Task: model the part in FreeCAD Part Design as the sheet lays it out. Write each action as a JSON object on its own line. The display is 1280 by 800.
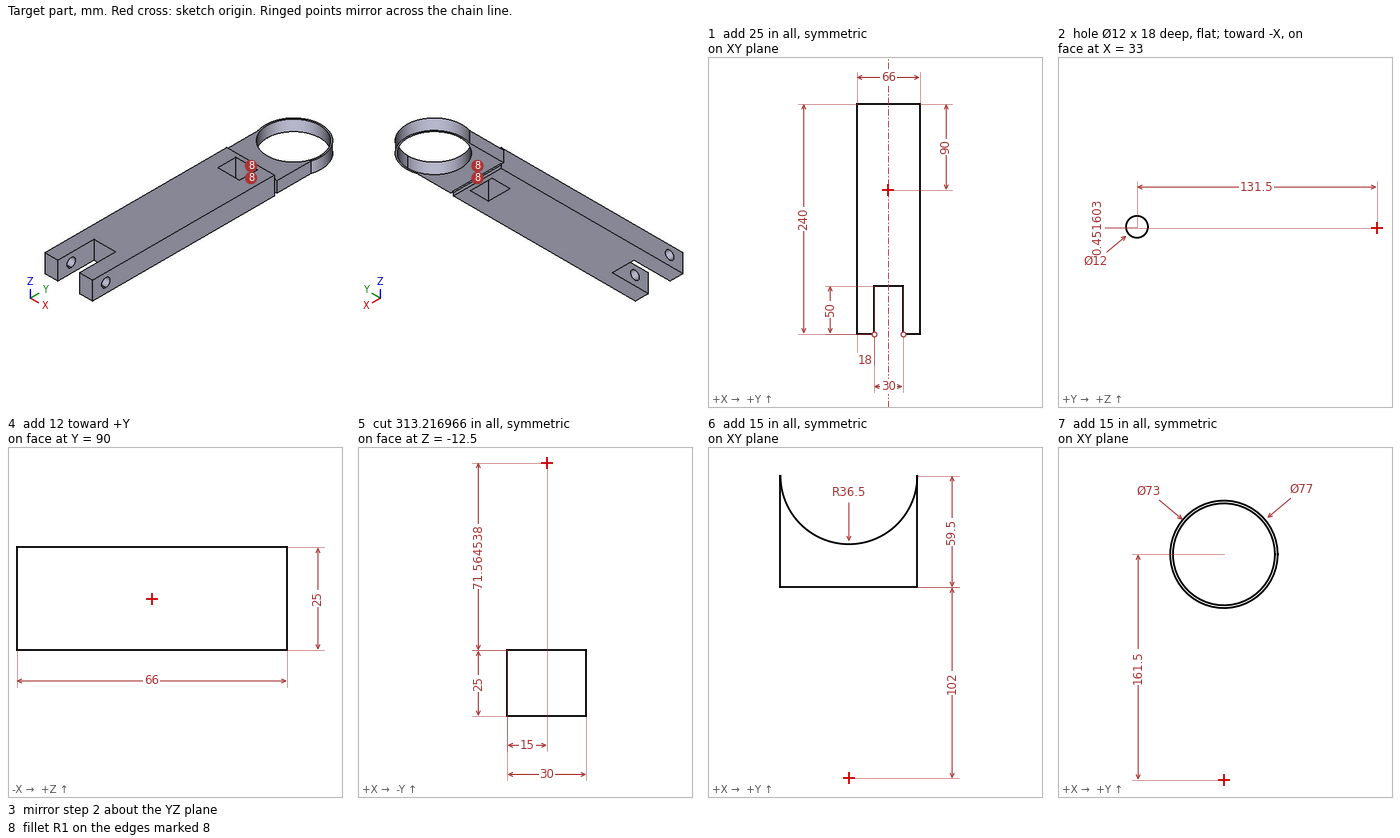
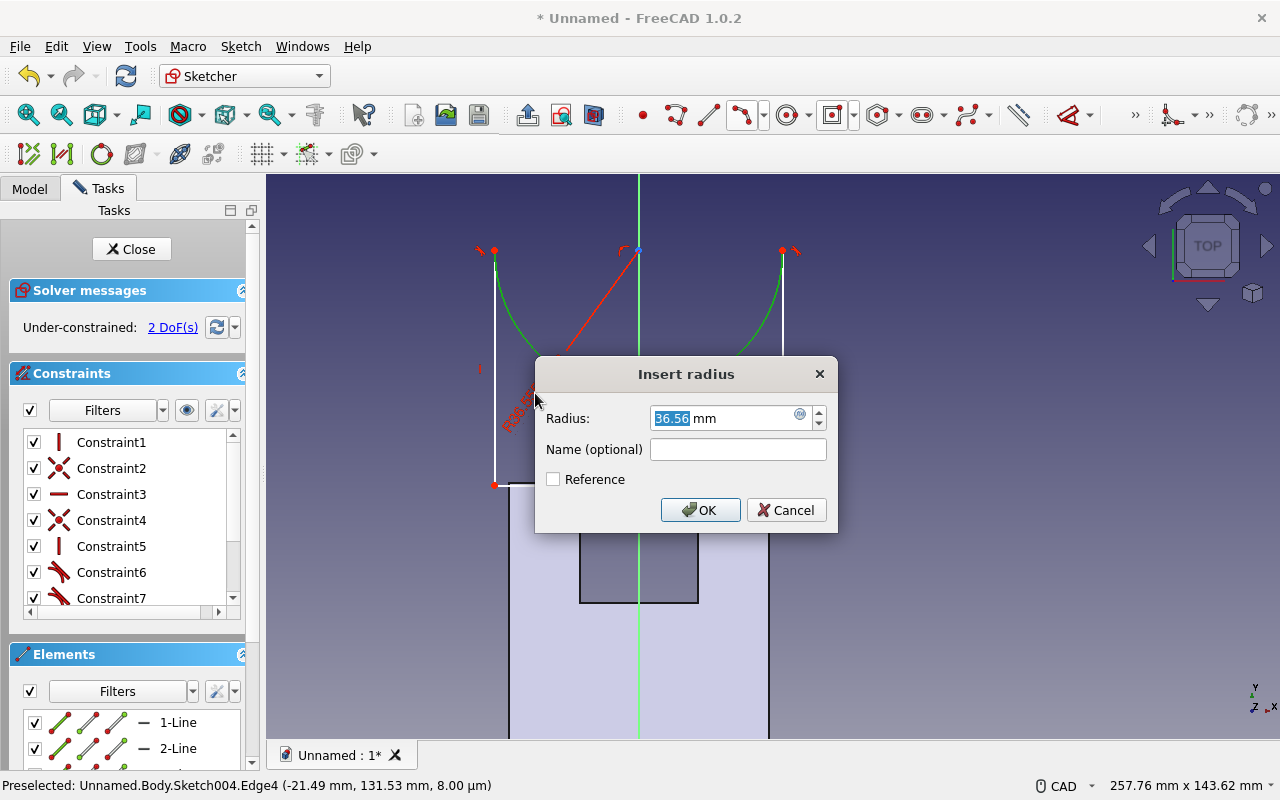
{"action": "type", "text": "36.5"}
{"action": "key", "text": "Return"}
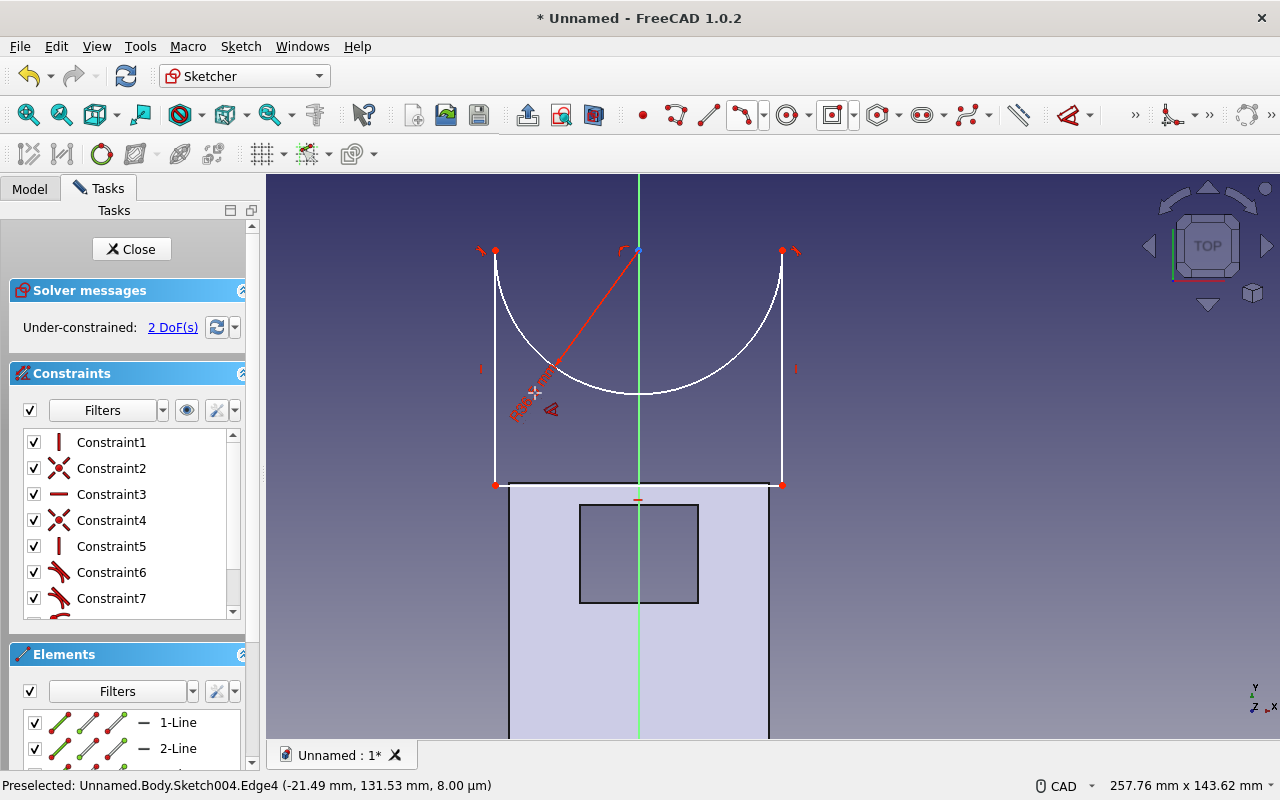
{"action": "left_click", "coordinate": [782, 321]}
{"action": "left_click", "coordinate": [816, 368]}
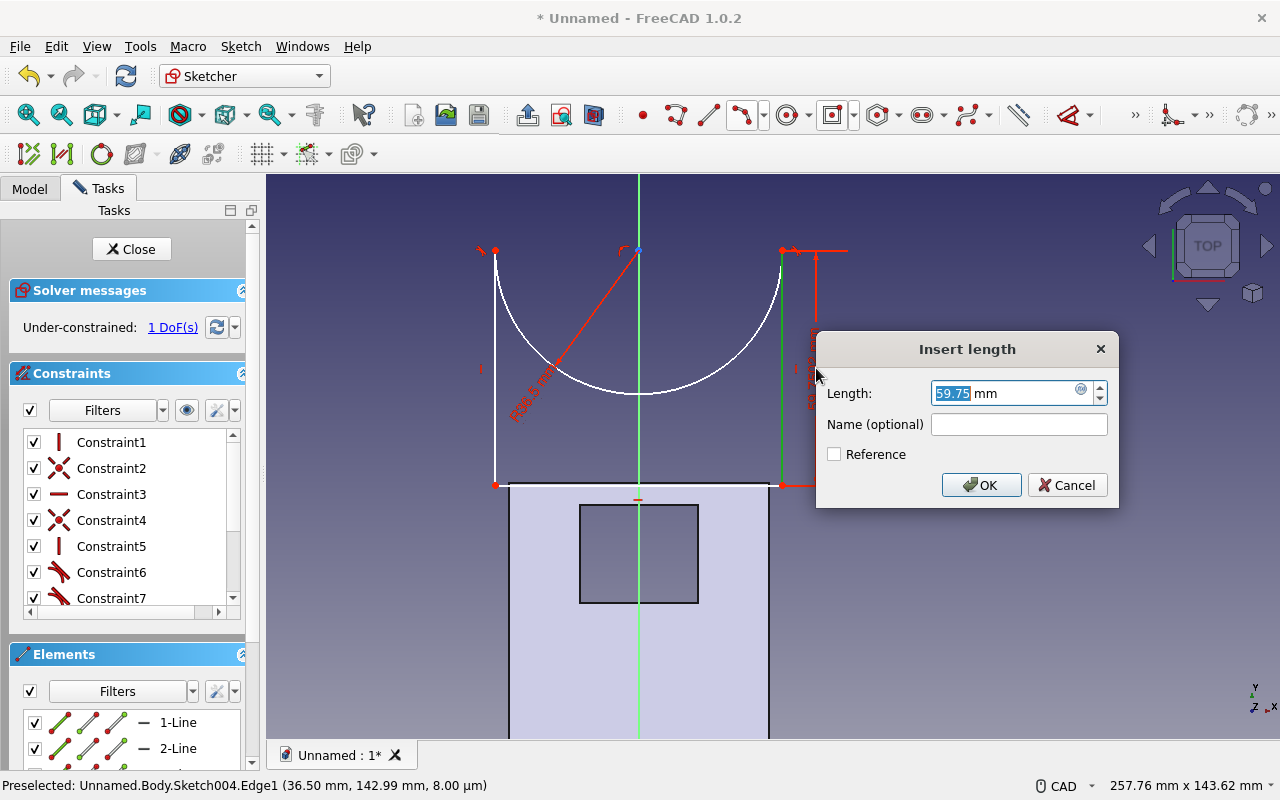
{"action": "type", "text": "59.5"}
{"action": "key", "text": "Return"}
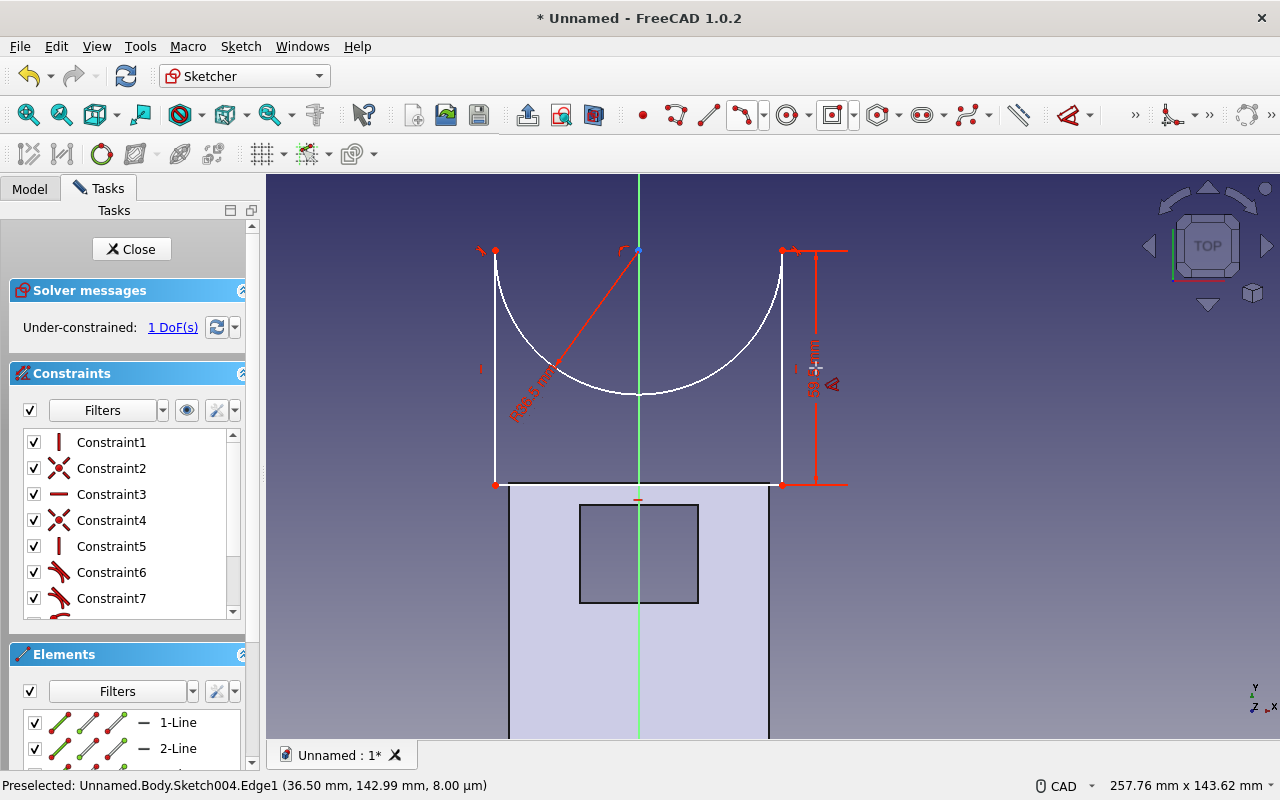
{"action": "left_click", "coordinate": [782, 485]}
{"action": "left_click", "coordinate": [816, 598]}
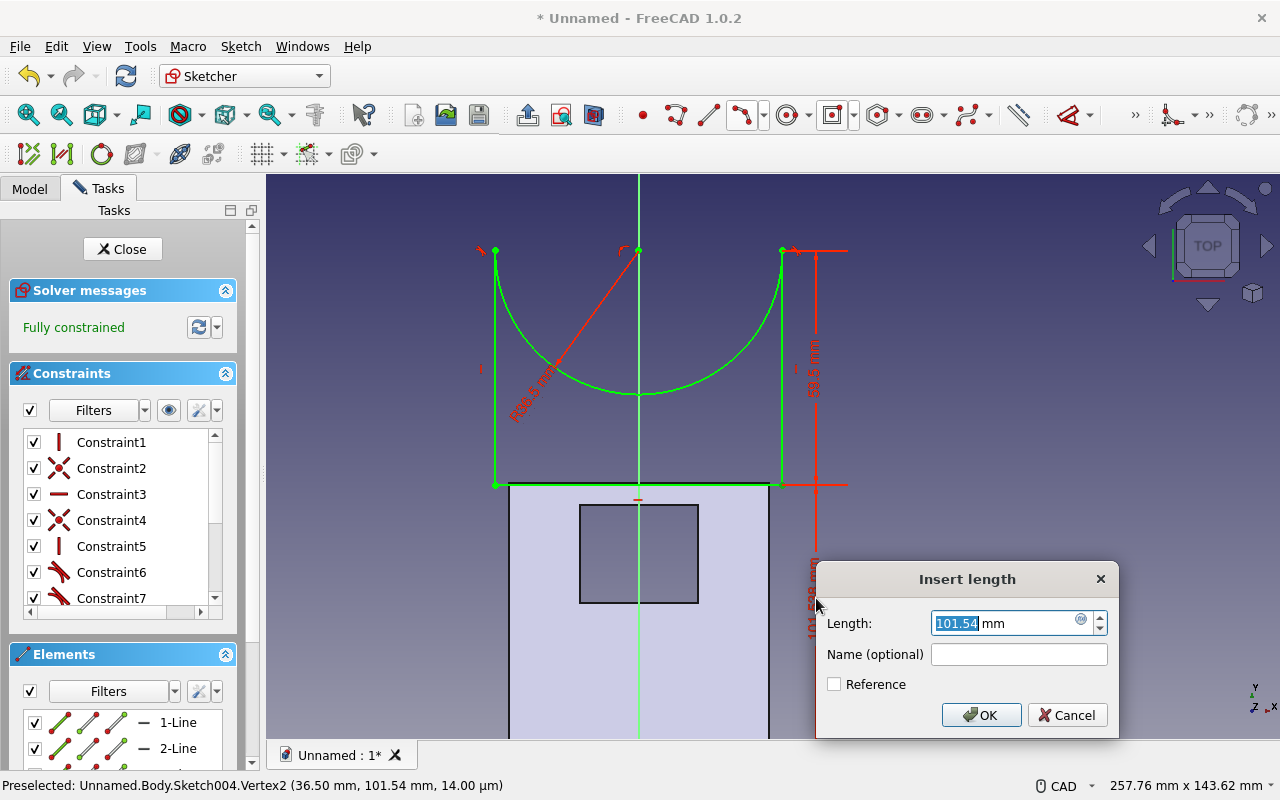
{"action": "type", "text": "102"}
{"action": "key", "text": "Return"}
{"action": "key", "text": "Escape"}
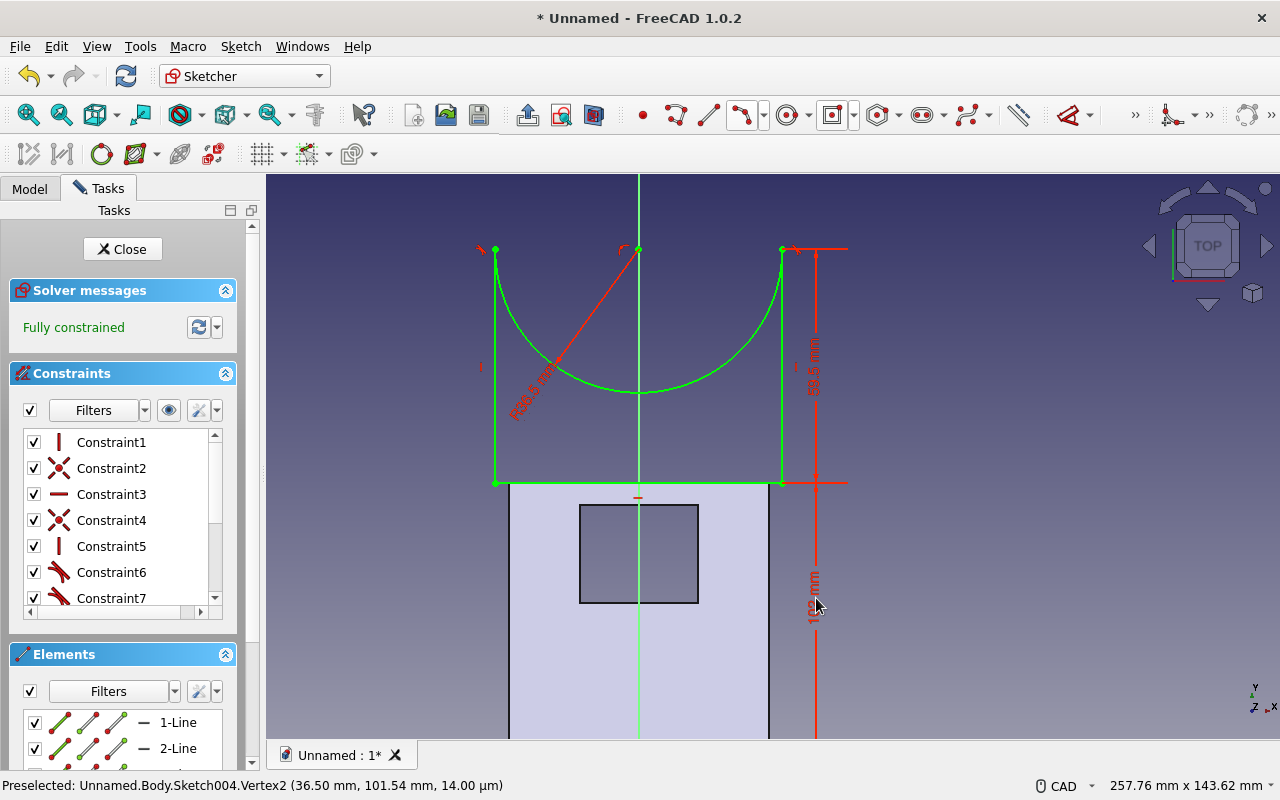
{"action": "left_click", "coordinate": [123, 249]}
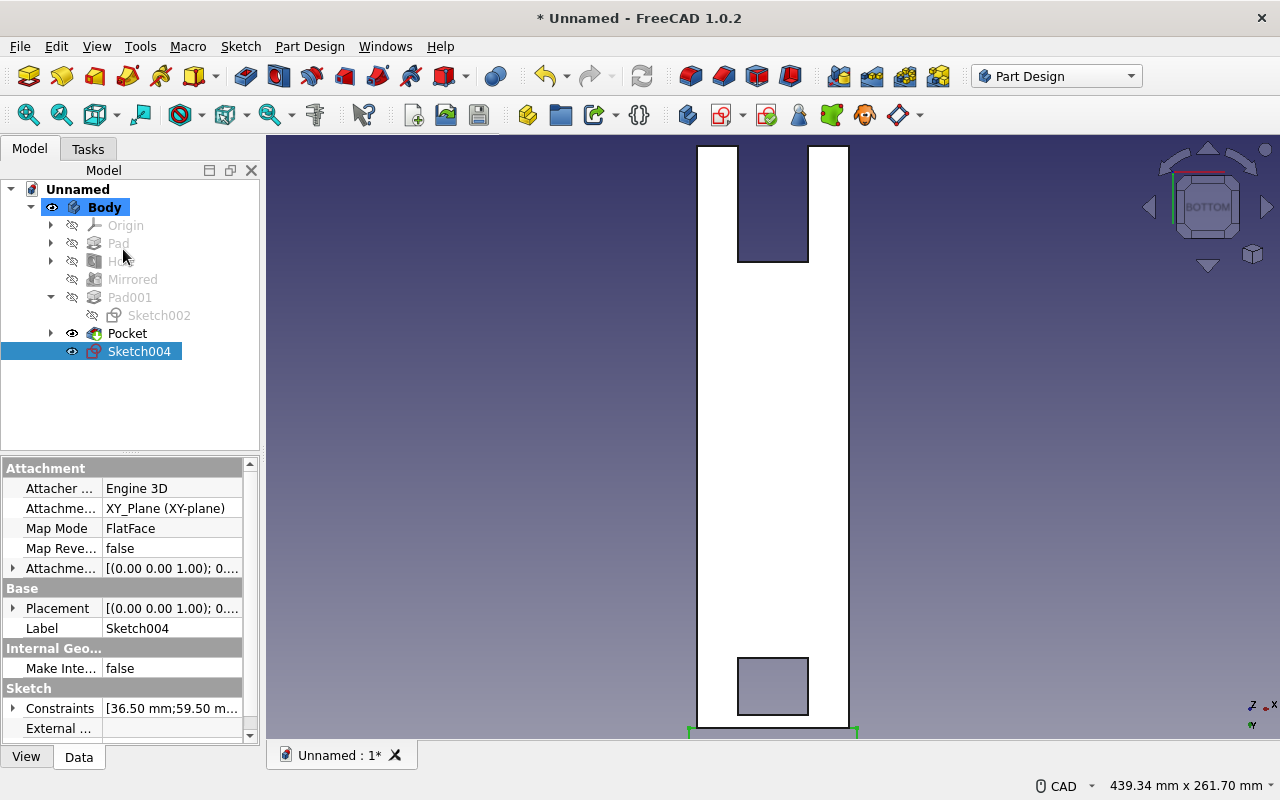
{"action": "left_click", "coordinate": [29, 76]}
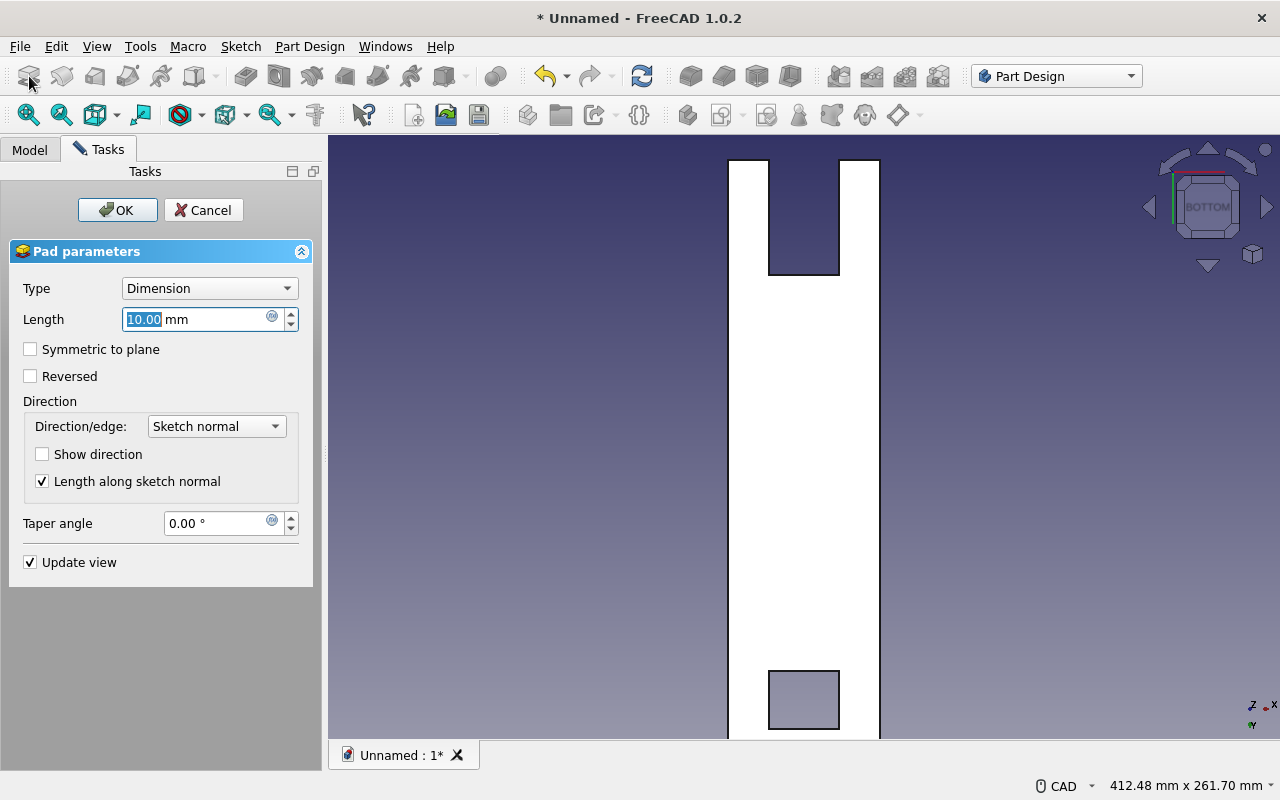
{"action": "type", "text": "15"}
{"action": "key", "text": "Tab"}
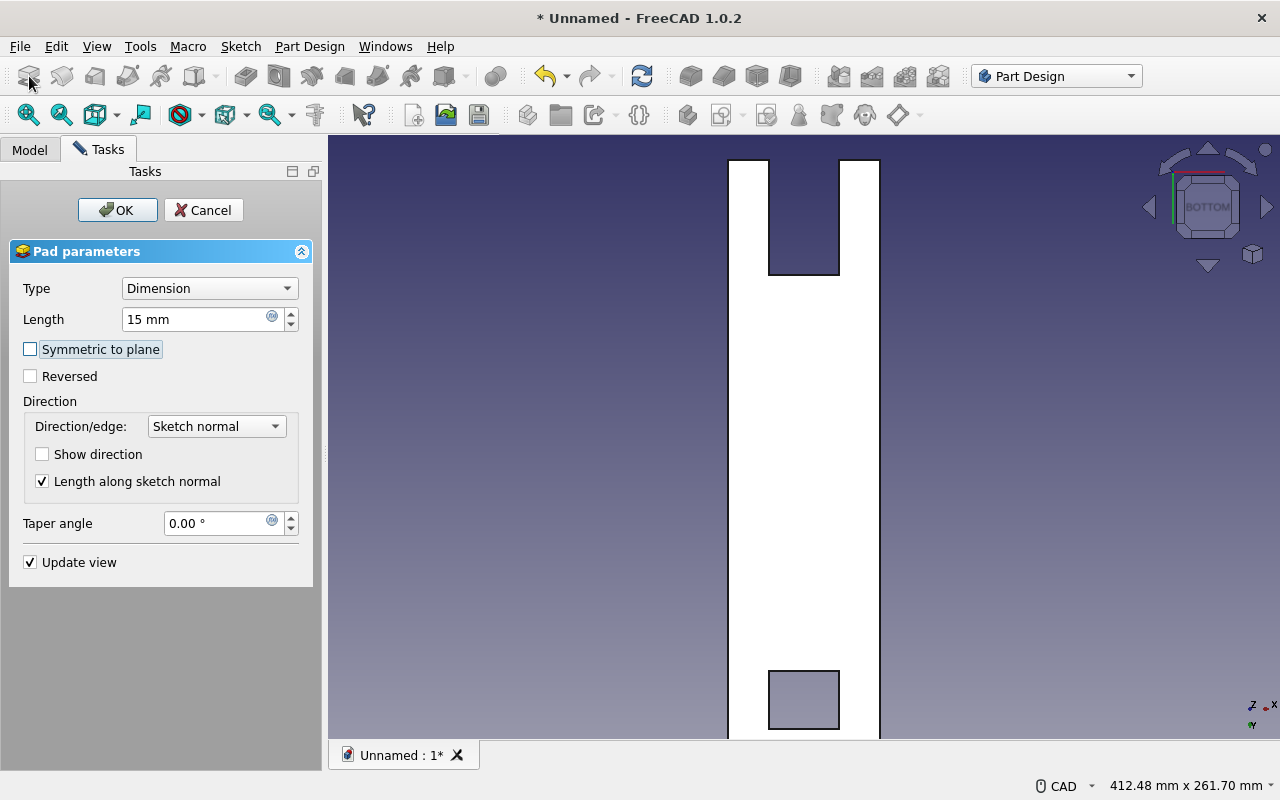
{"action": "left_click", "coordinate": [31, 349]}